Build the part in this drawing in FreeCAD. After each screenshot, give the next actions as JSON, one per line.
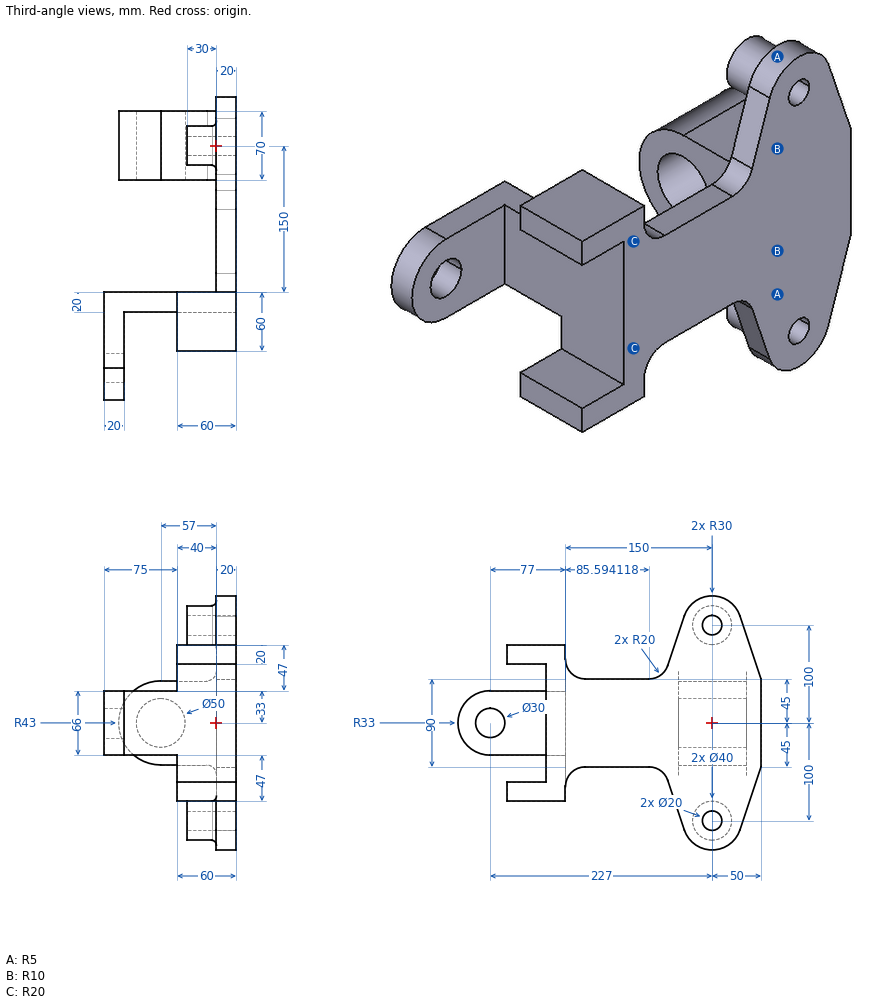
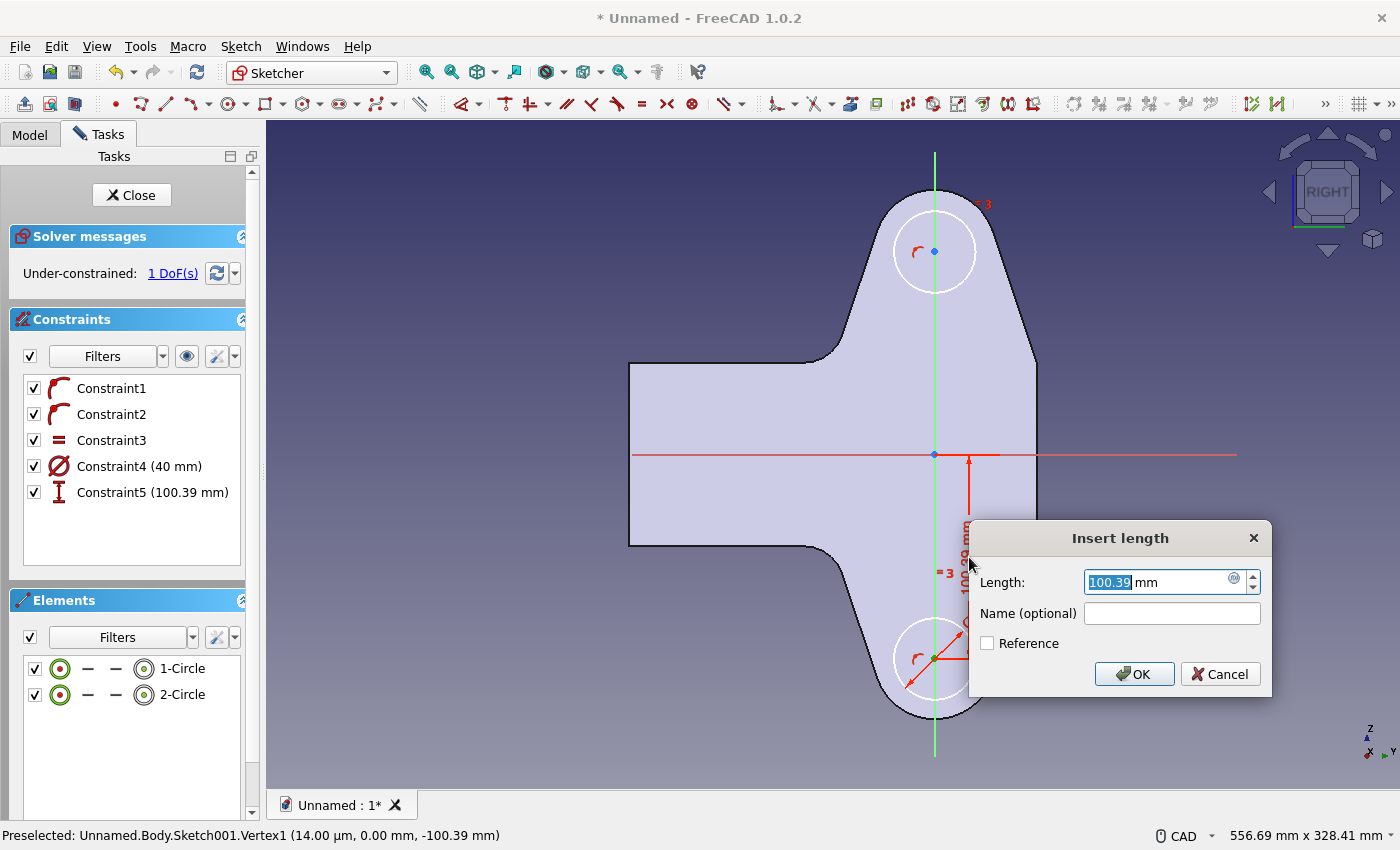
{"action": "type", "text": "100"}
{"action": "key", "text": "Return"}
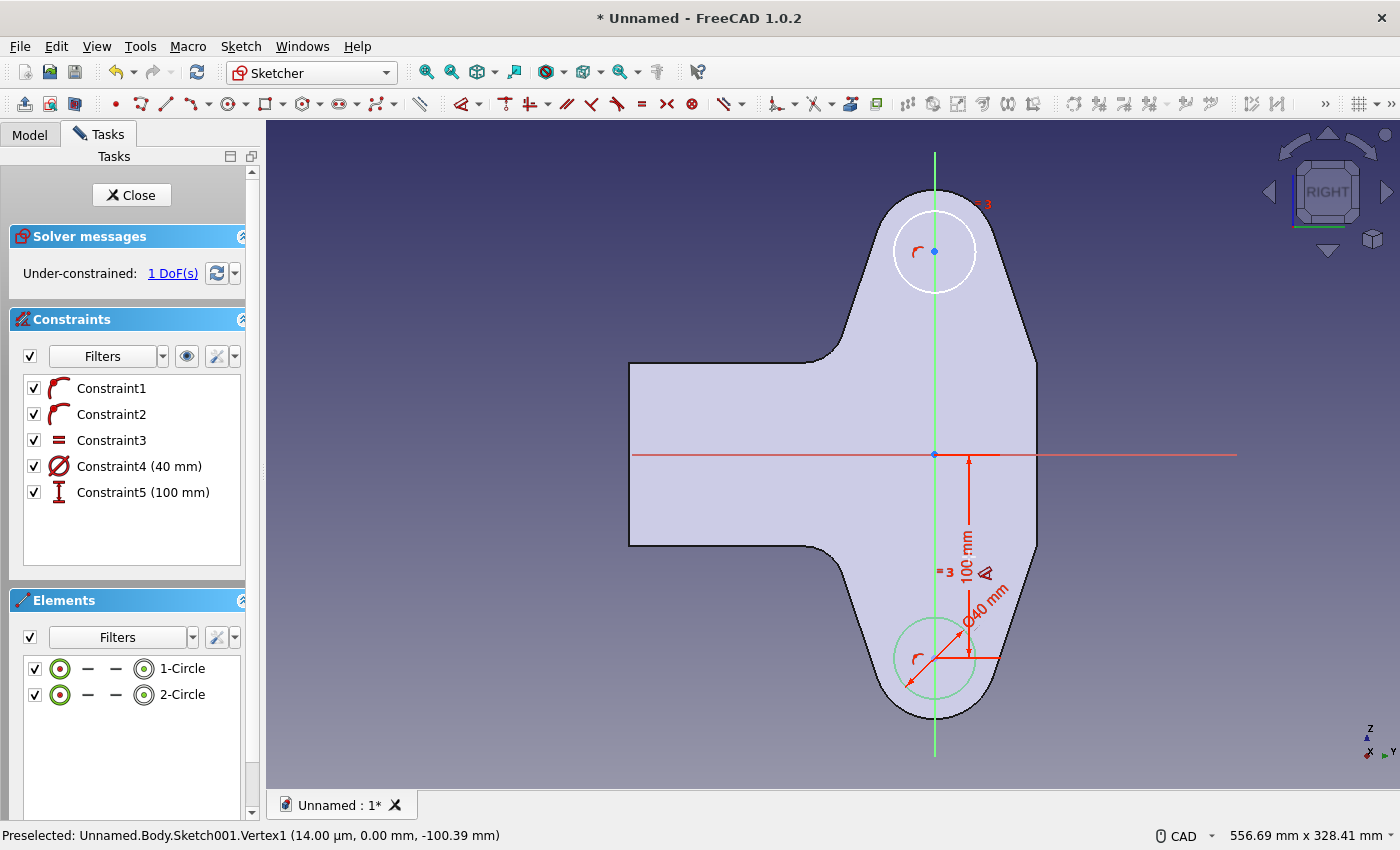
{"action": "left_click", "coordinate": [935, 252]}
{"action": "left_click", "coordinate": [969, 353]}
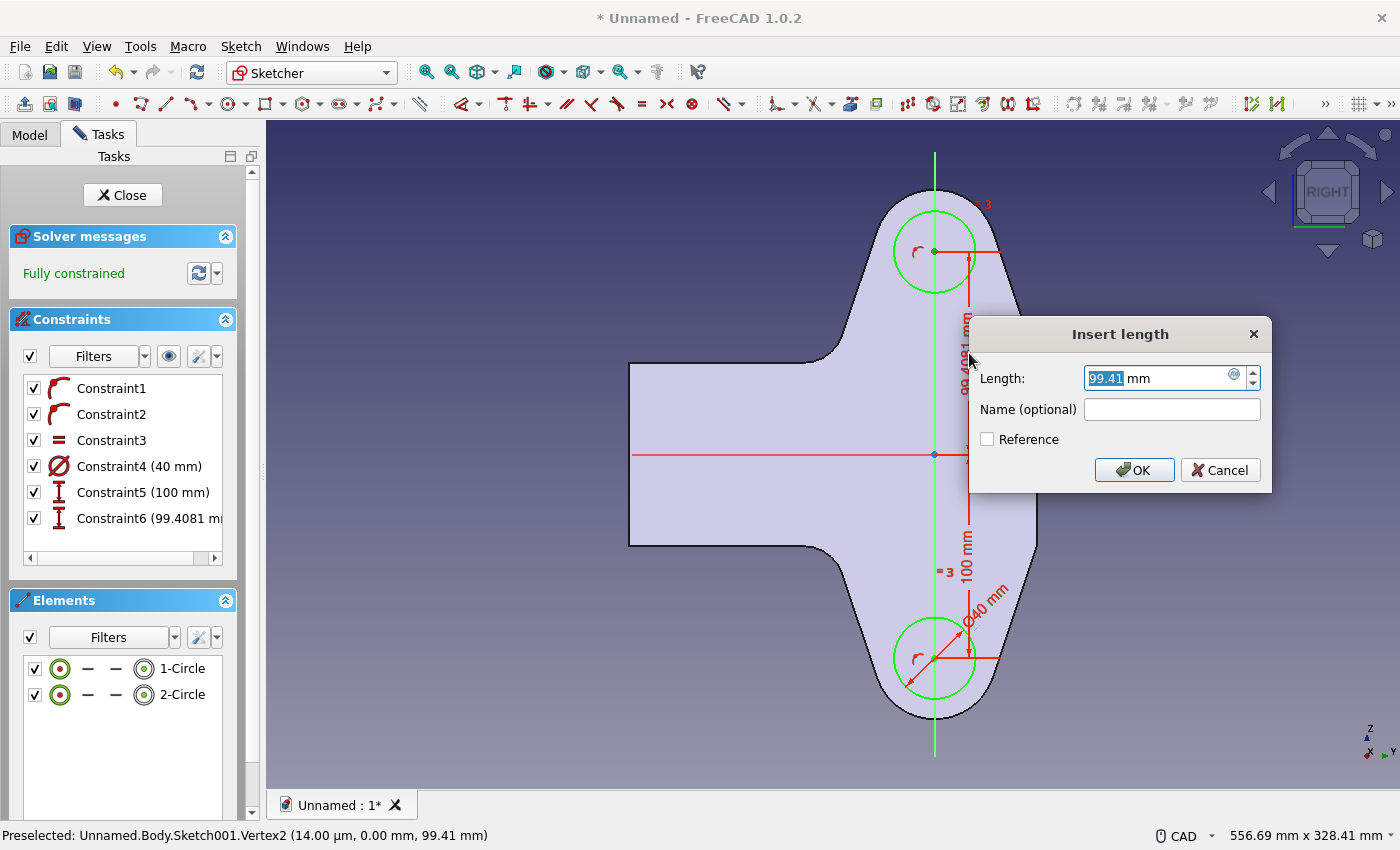
{"action": "type", "text": "100"}
{"action": "key", "text": "Return"}
{"action": "key", "text": "Escape"}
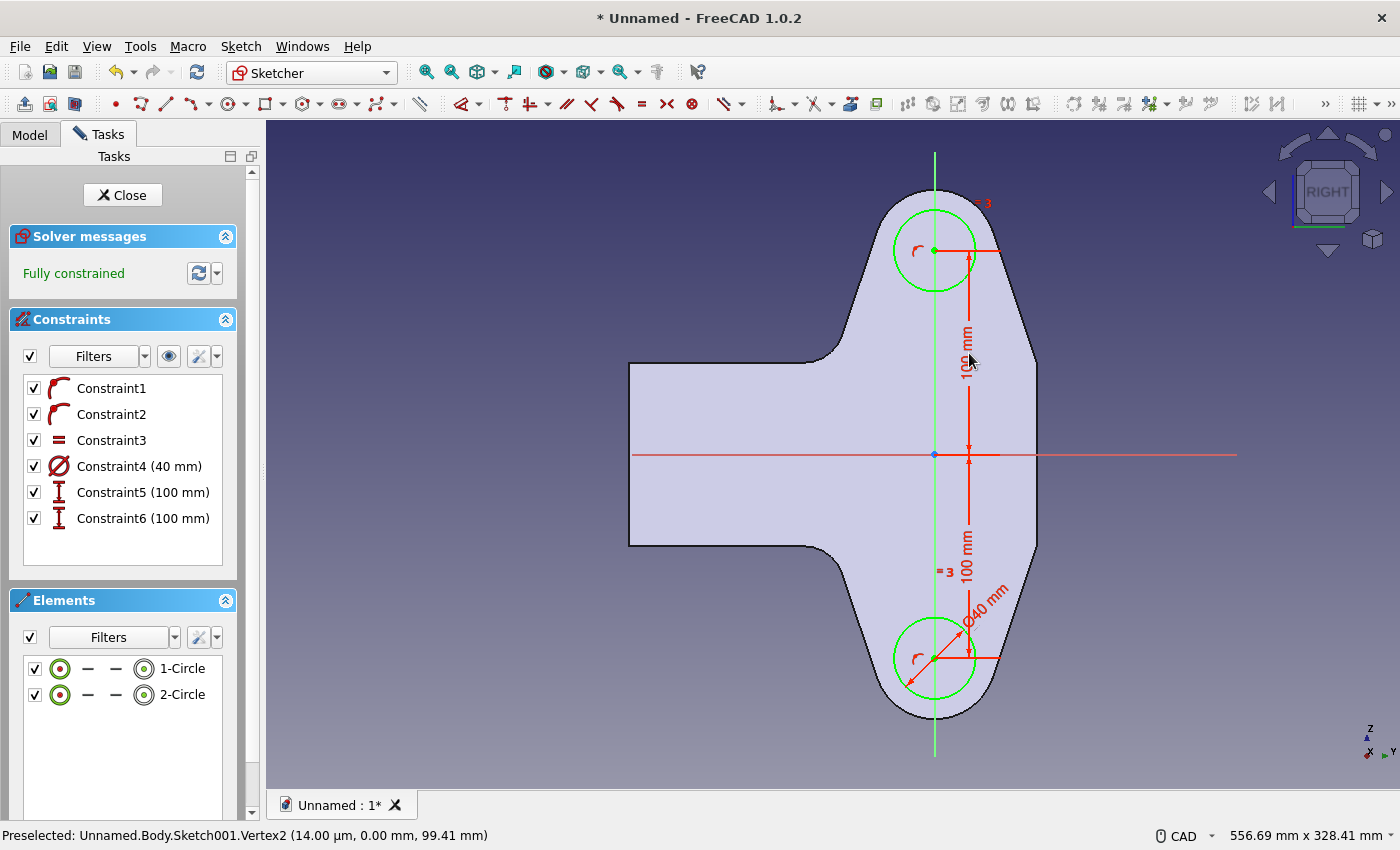
{"action": "left_click", "coordinate": [123, 195]}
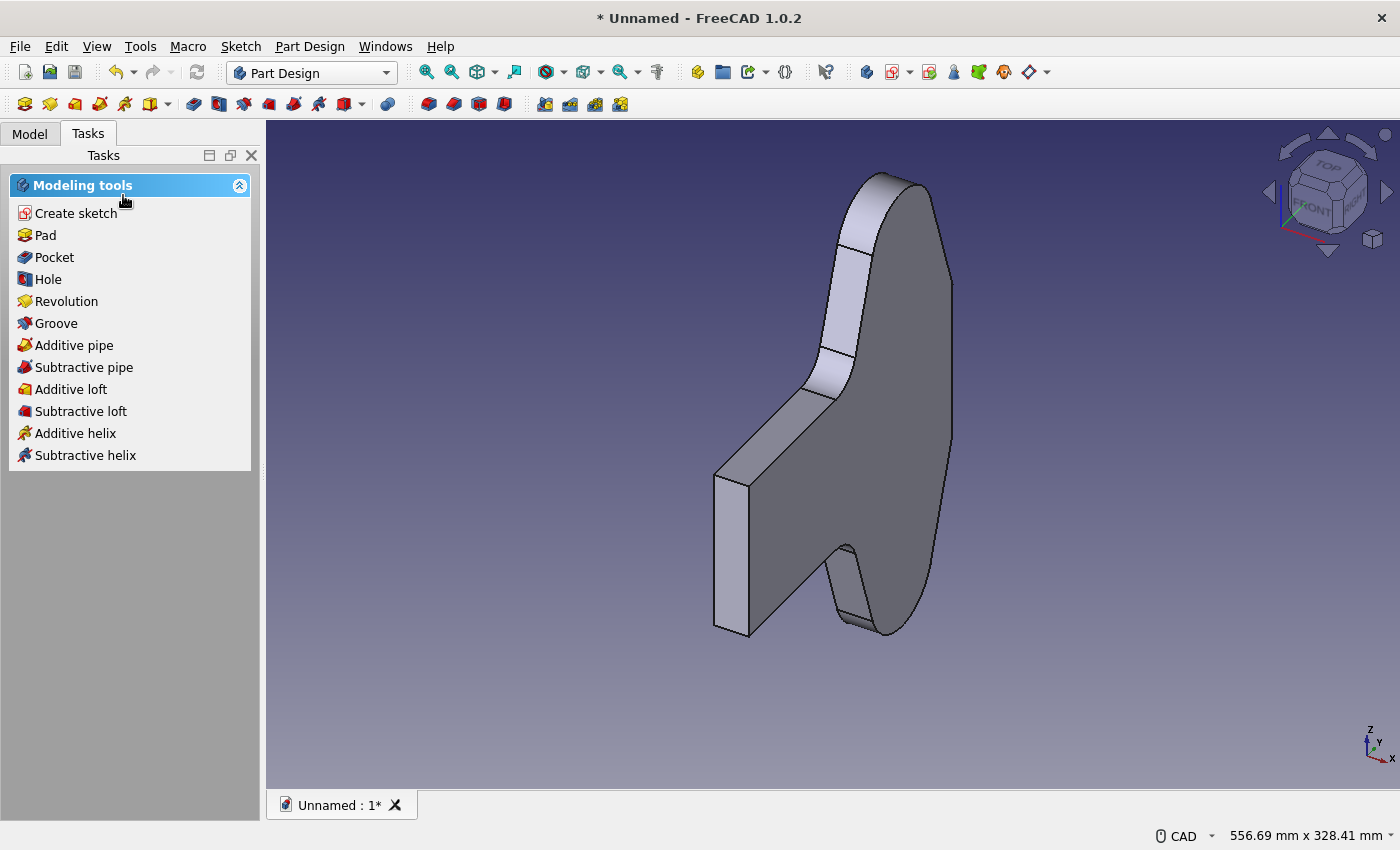
{"action": "left_click", "coordinate": [25, 104]}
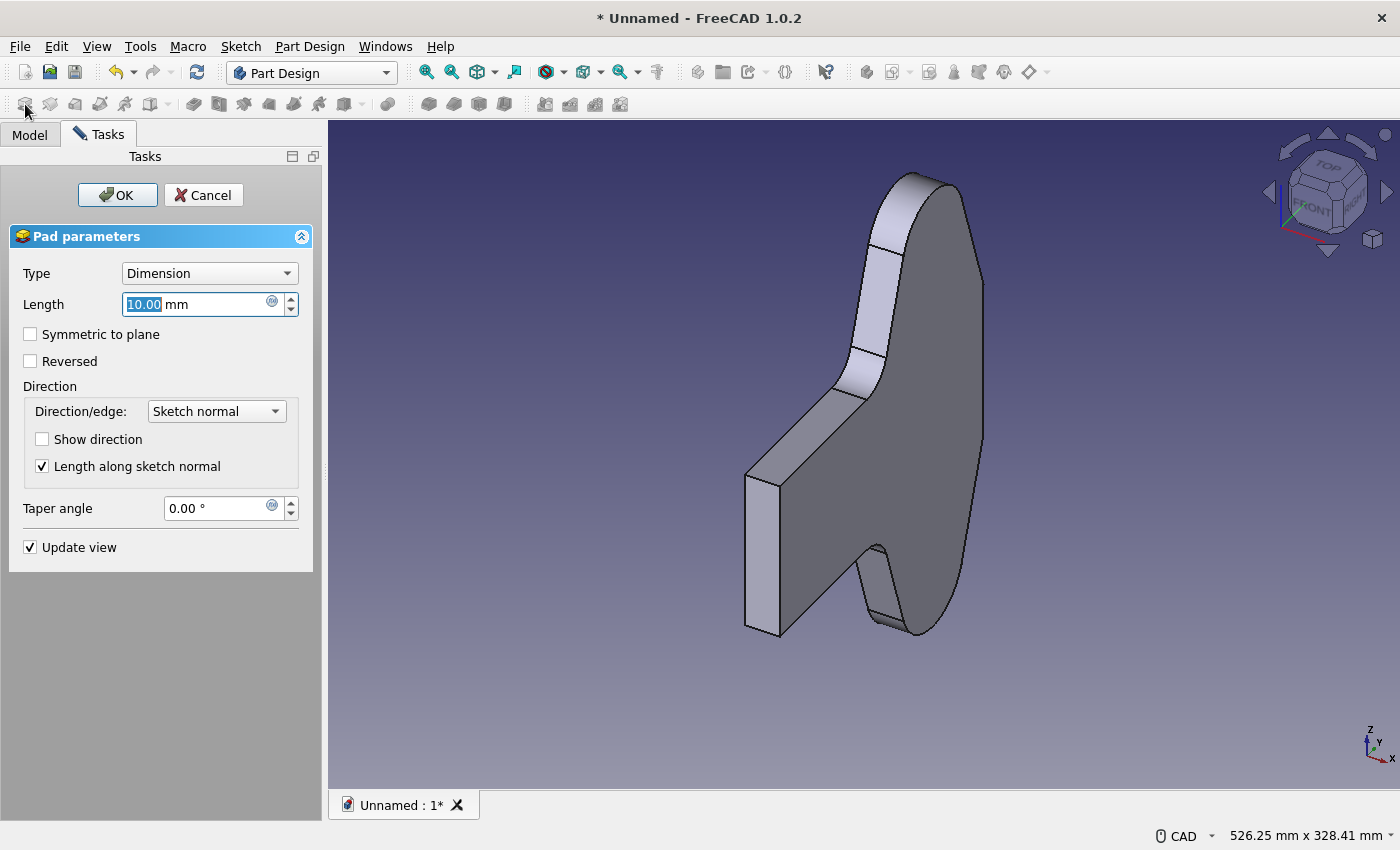
{"action": "type", "text": "30"}
{"action": "key", "text": "Tab"}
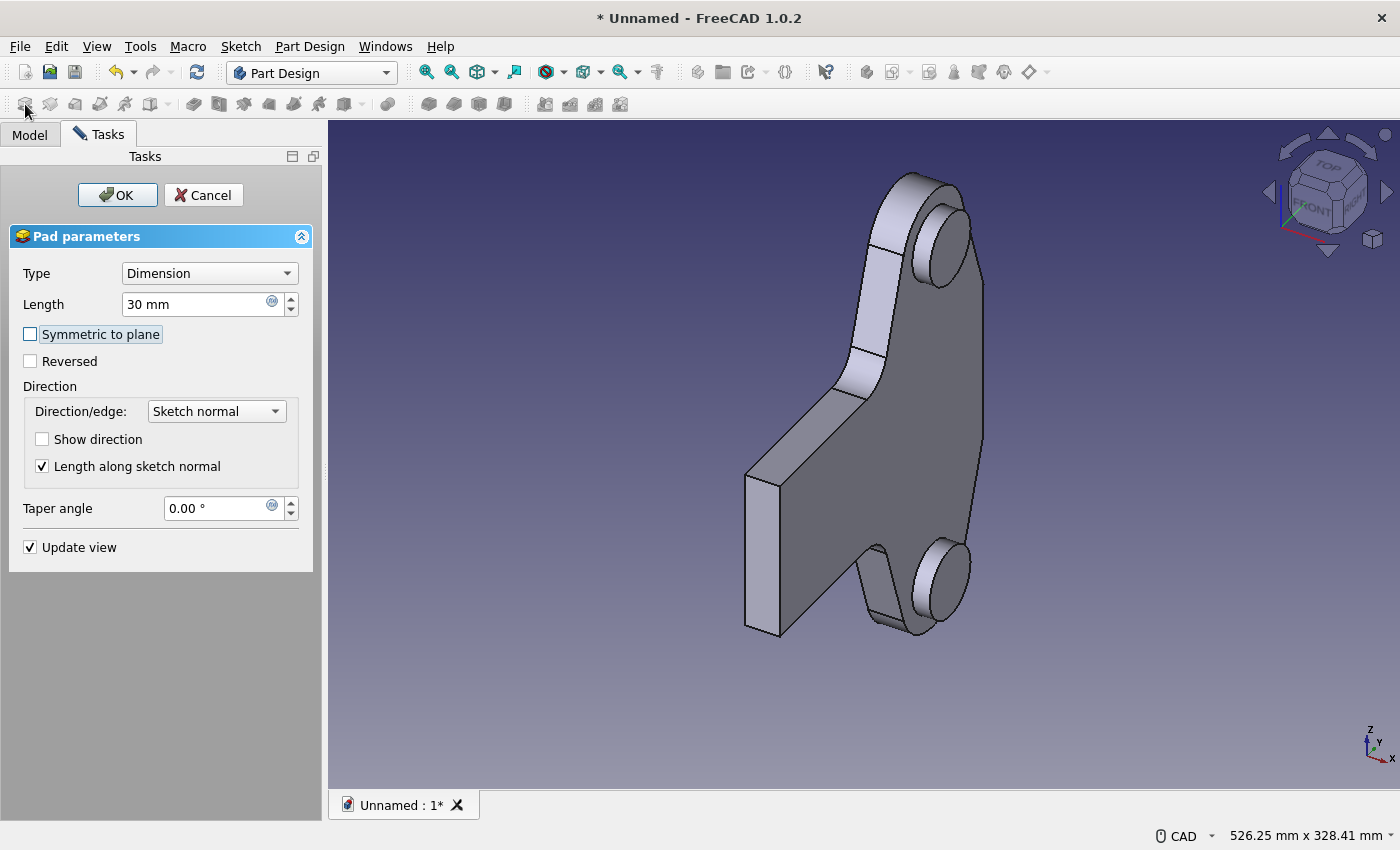
{"action": "left_click", "coordinate": [31, 361]}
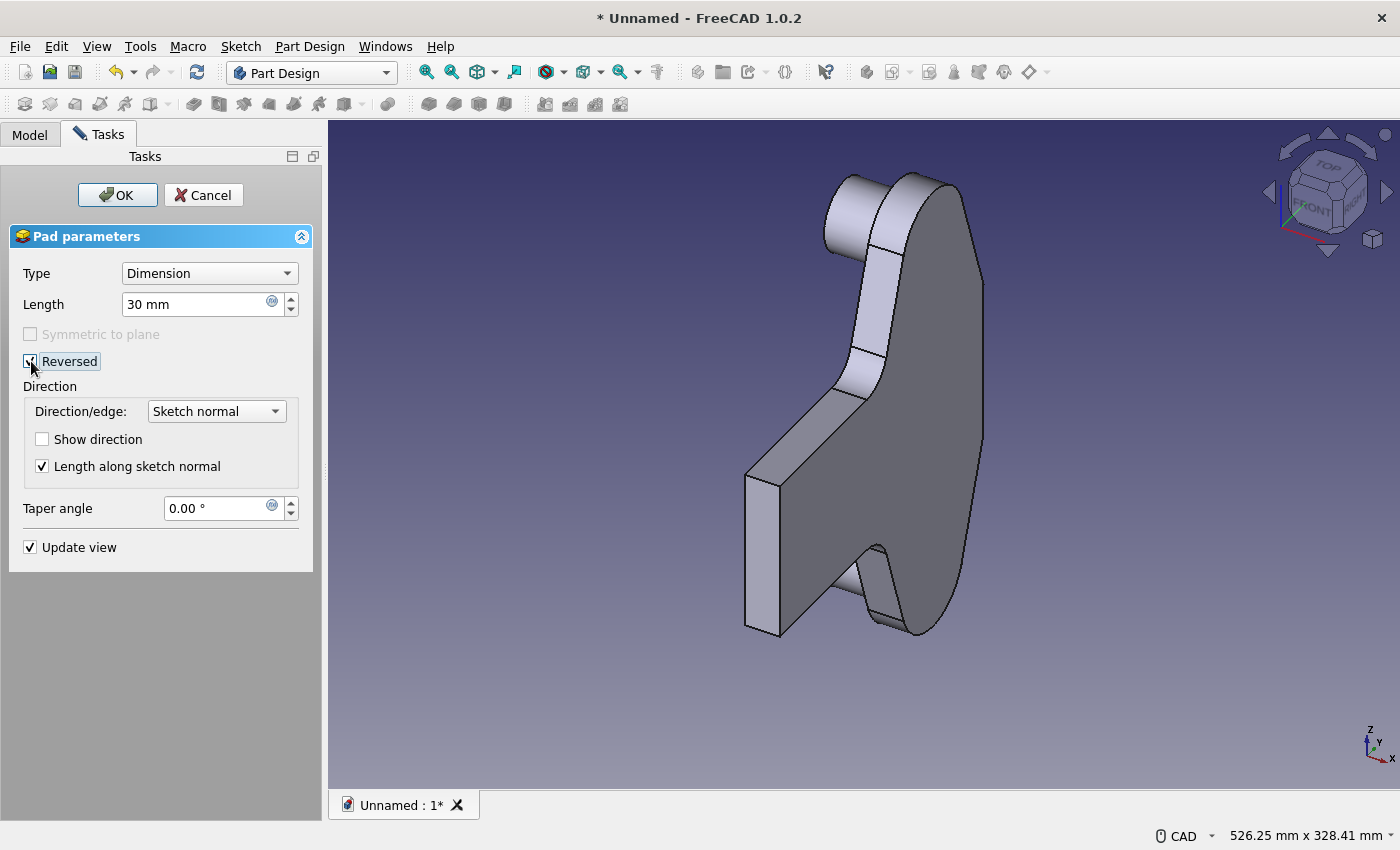
{"action": "left_click", "coordinate": [118, 195]}